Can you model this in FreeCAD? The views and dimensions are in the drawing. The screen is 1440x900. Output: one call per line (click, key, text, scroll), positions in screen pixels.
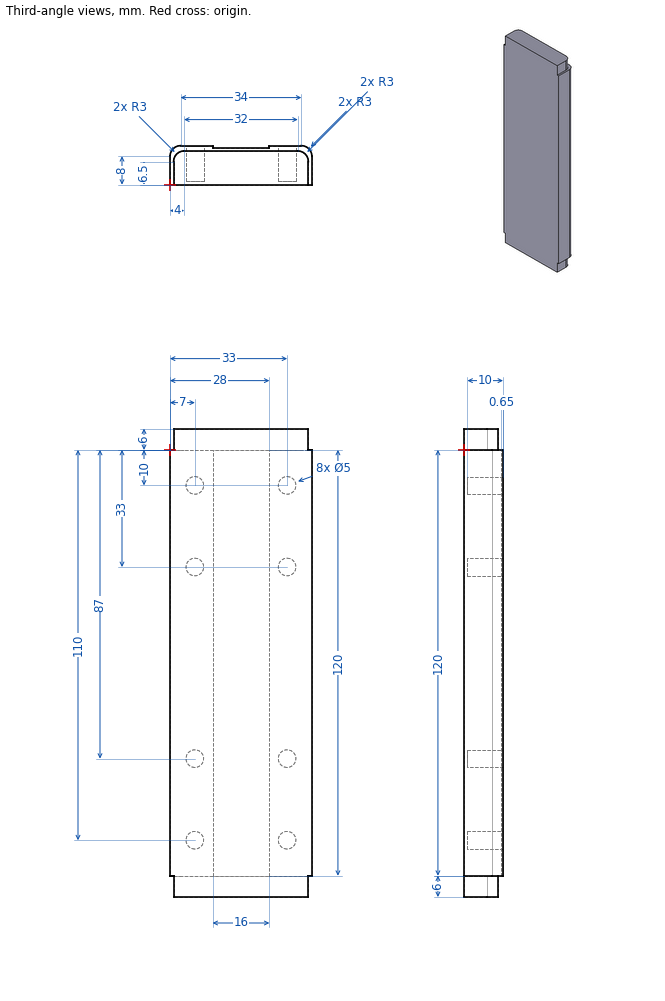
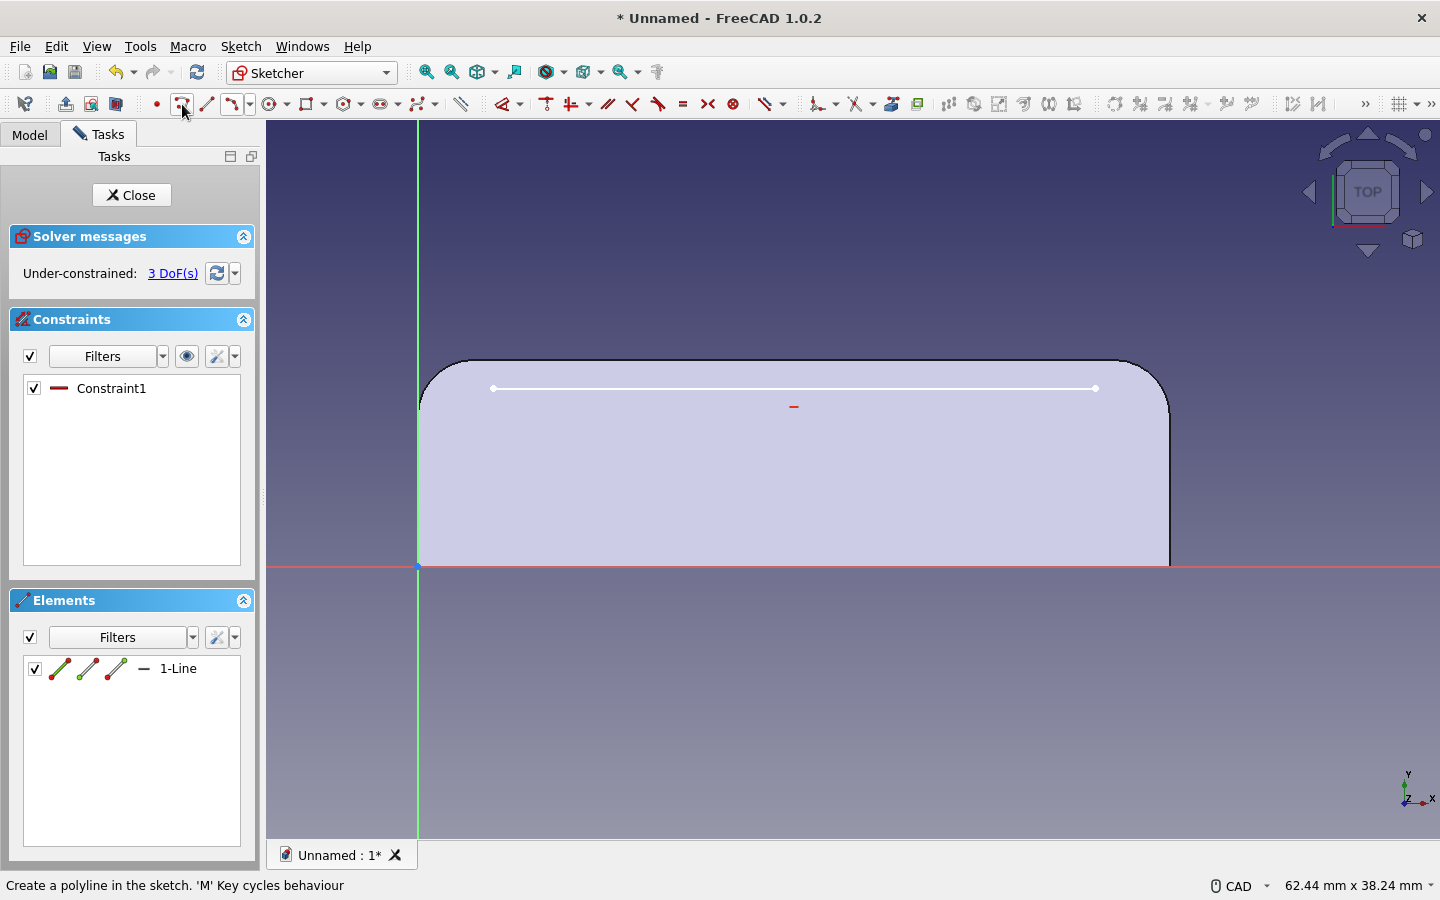
click(437, 444)
click(437, 567)
click(1151, 558)
click(1151, 444)
right_click(1151, 444)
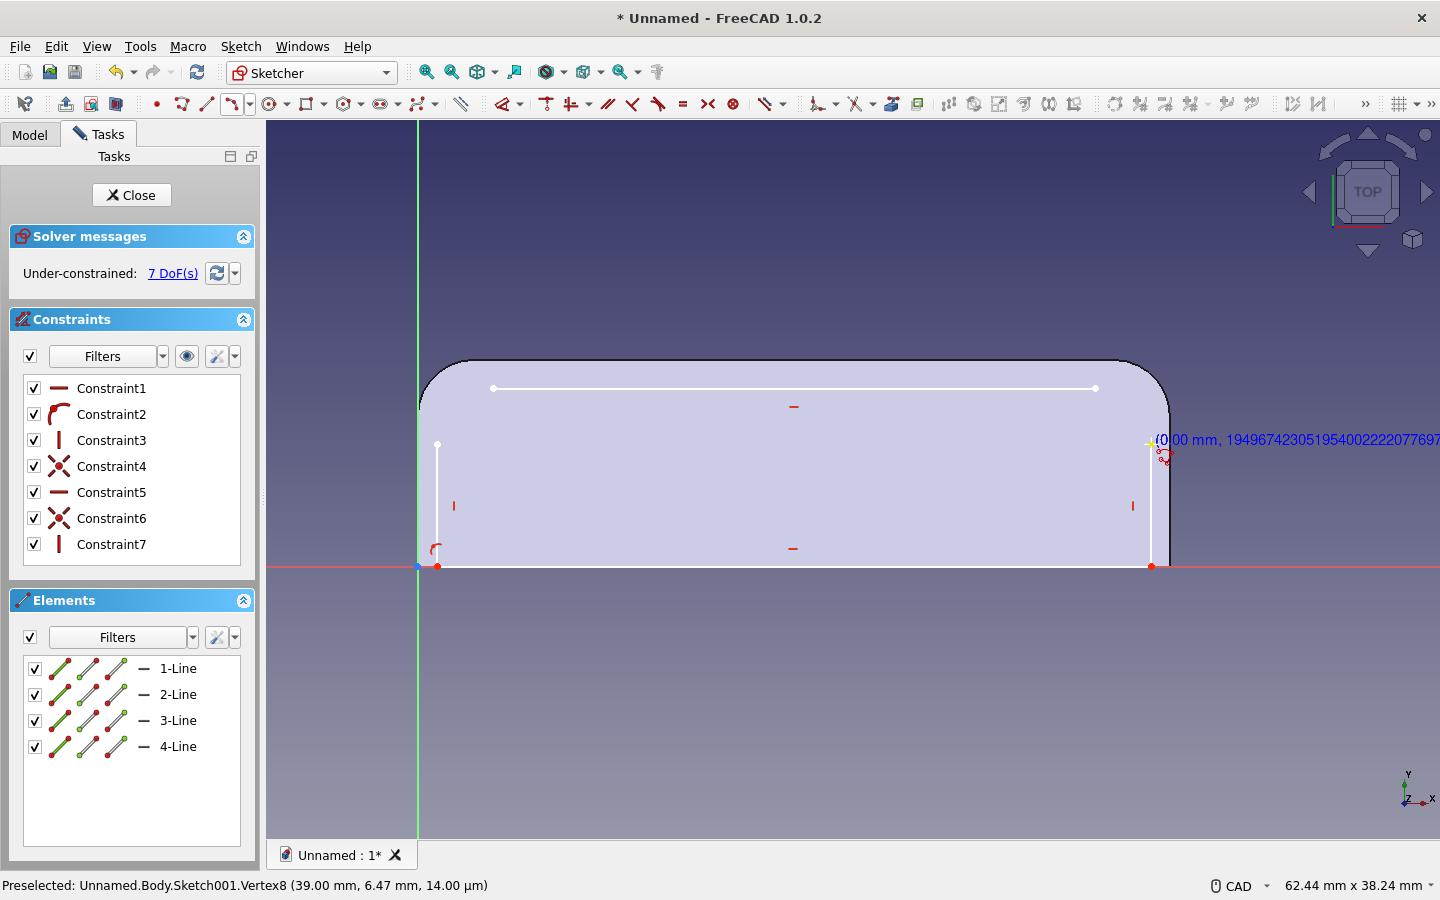
click(232, 104)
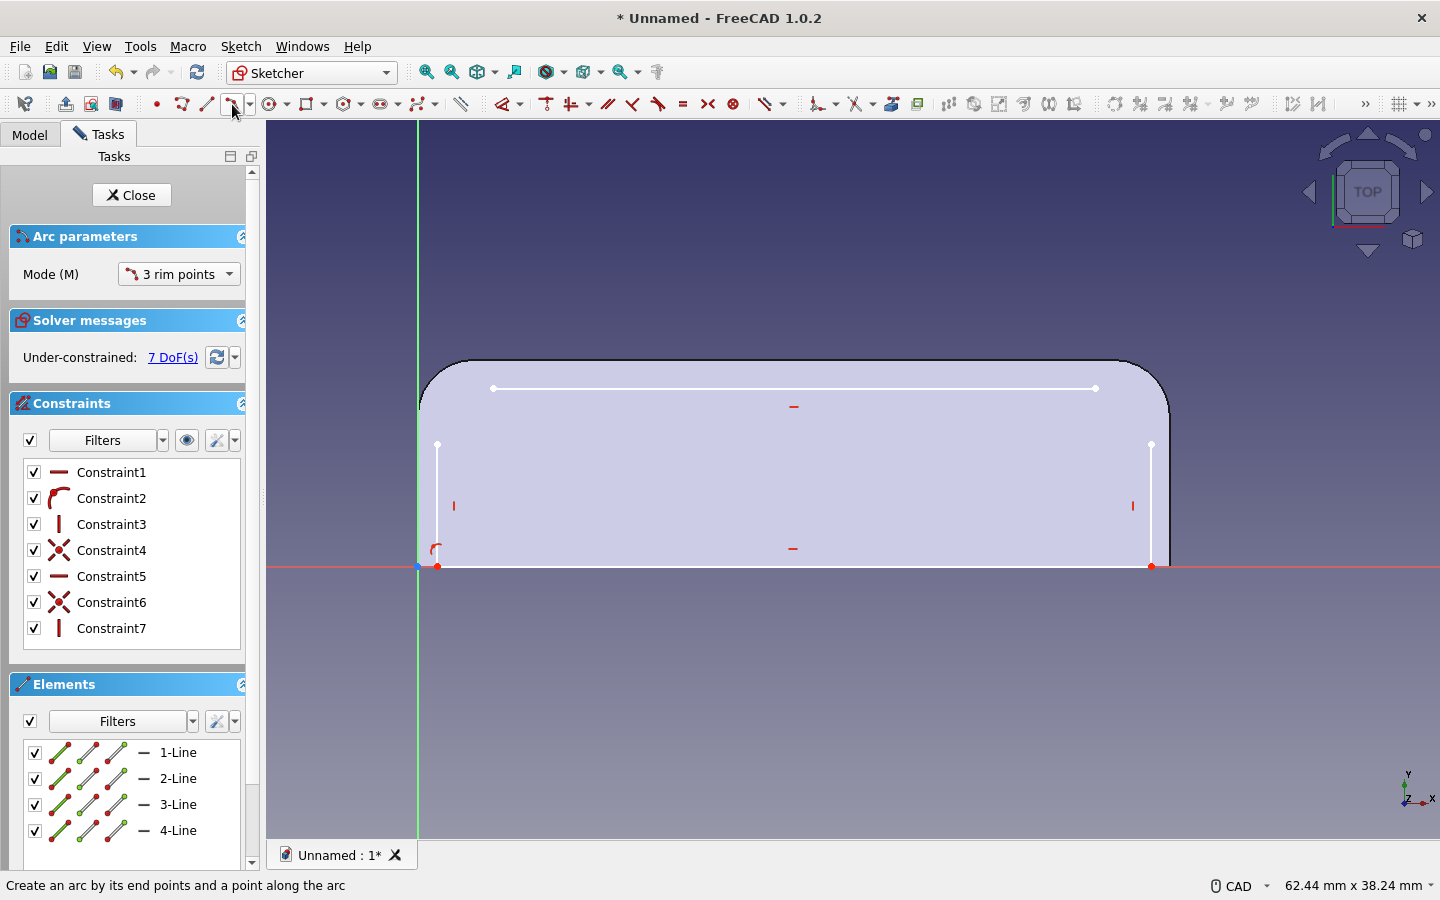
click(493, 389)
click(437, 445)
click(453, 405)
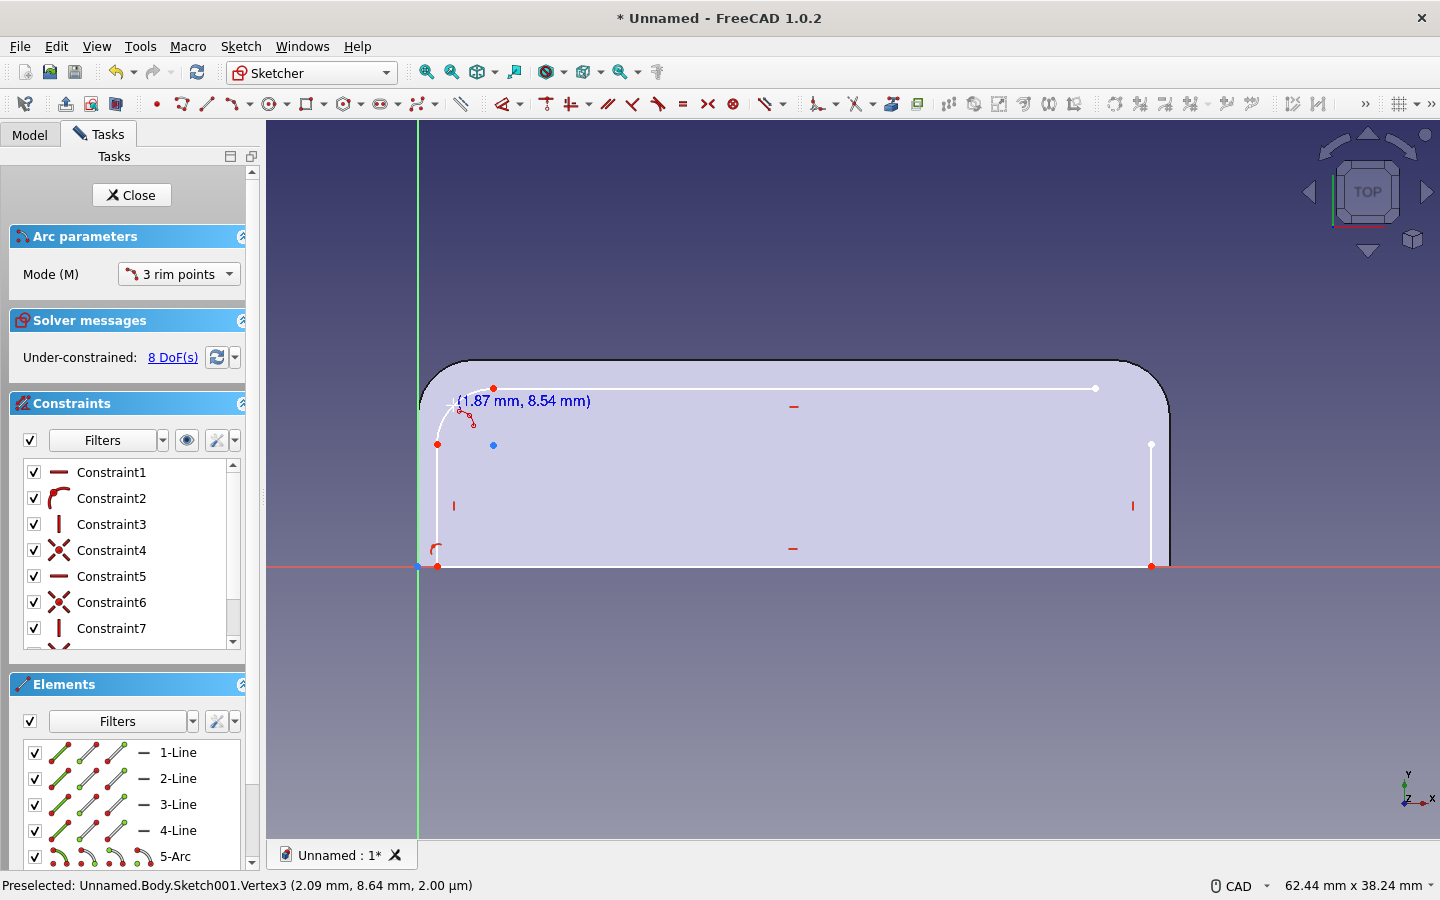
click(1151, 445)
click(1095, 389)
click(1134, 405)
key(Escape)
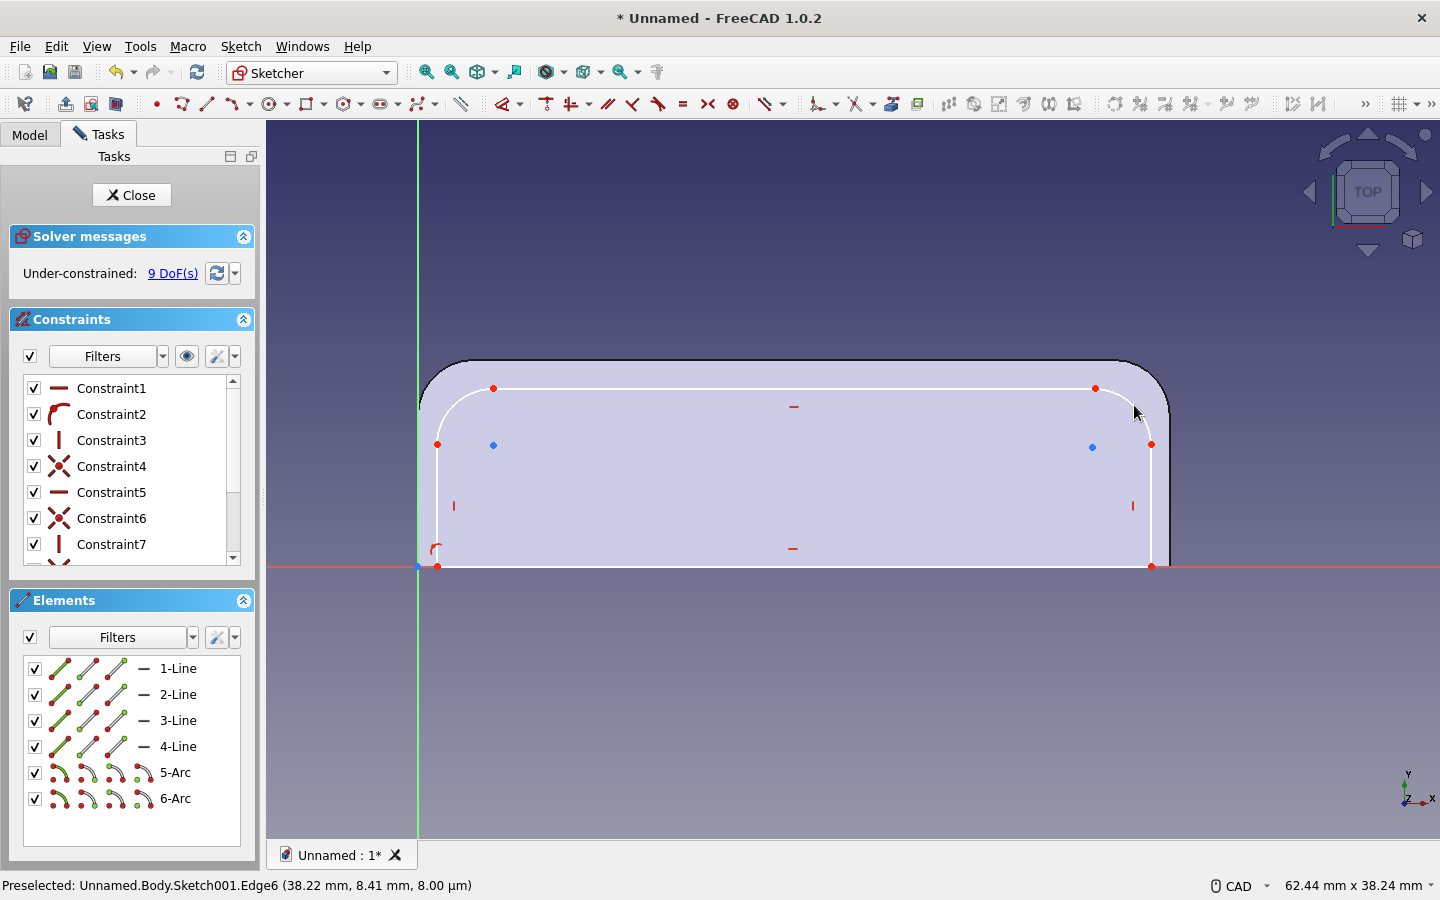
click(914, 389)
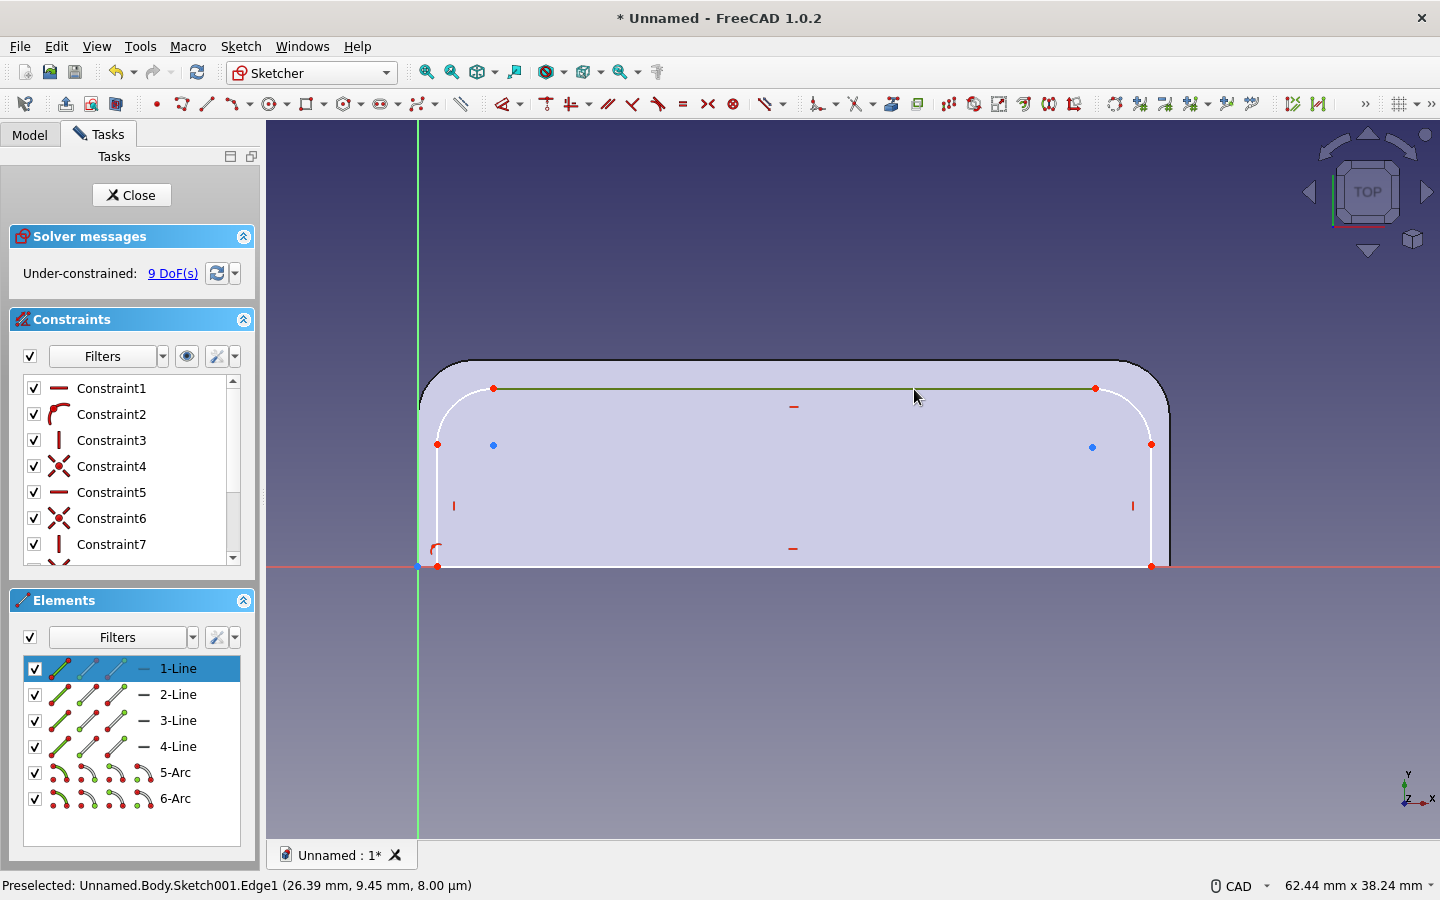
click(468, 395)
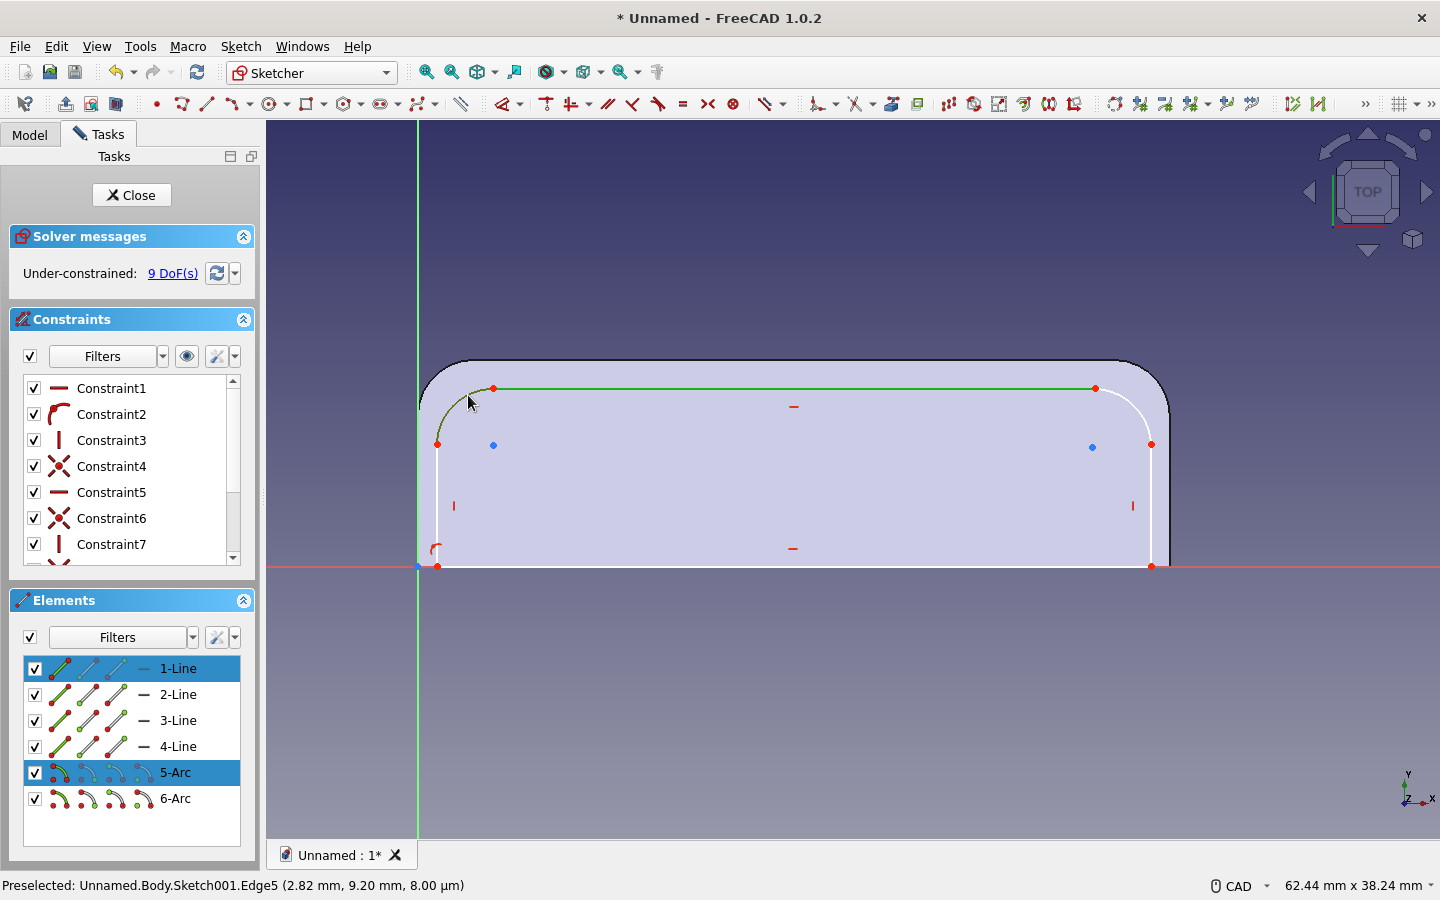
click(658, 104)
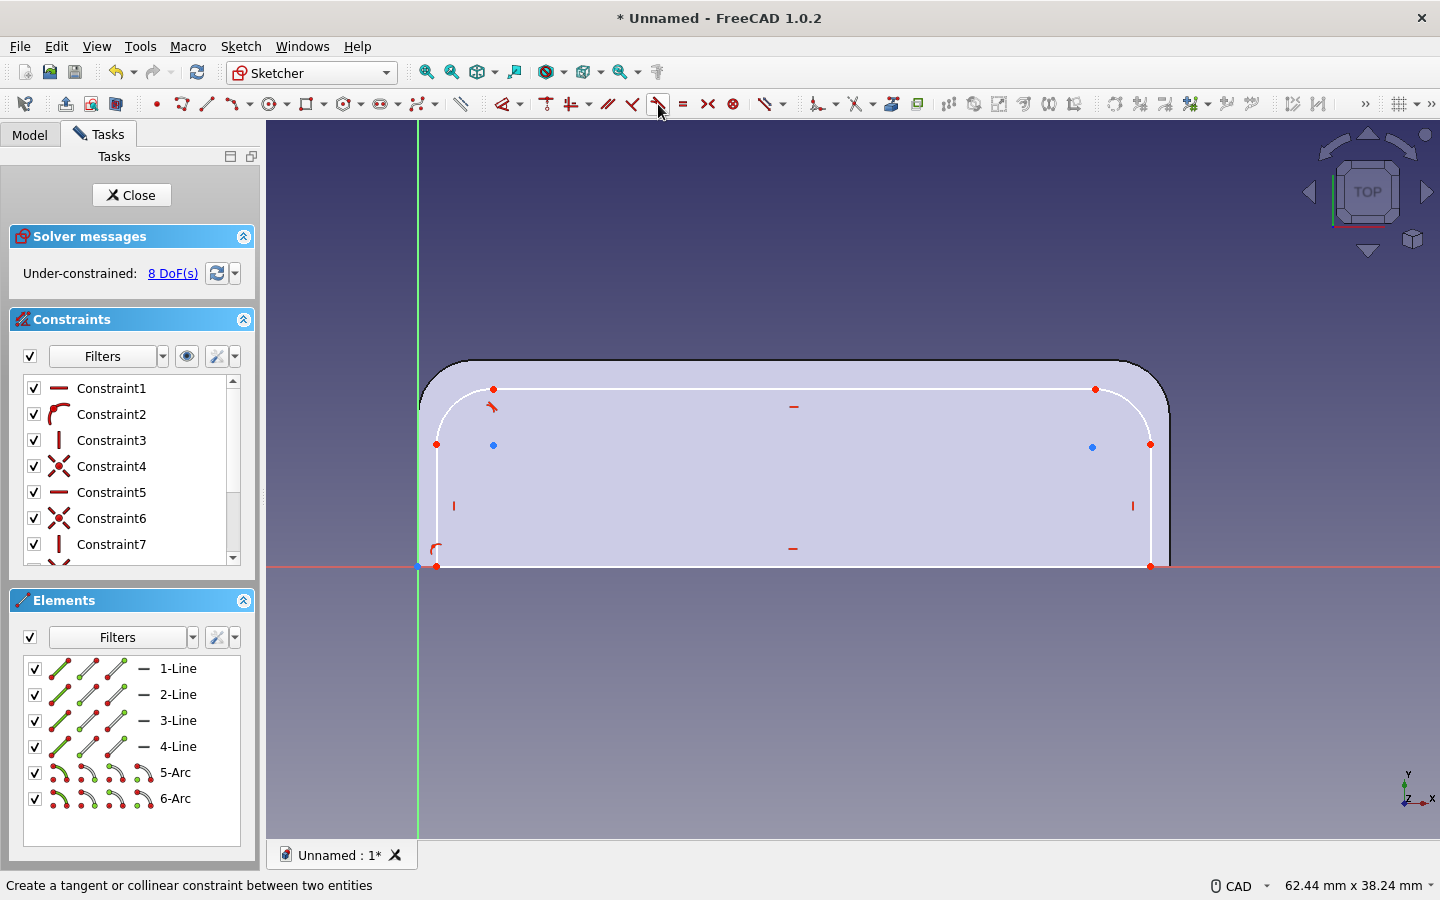
click(914, 389)